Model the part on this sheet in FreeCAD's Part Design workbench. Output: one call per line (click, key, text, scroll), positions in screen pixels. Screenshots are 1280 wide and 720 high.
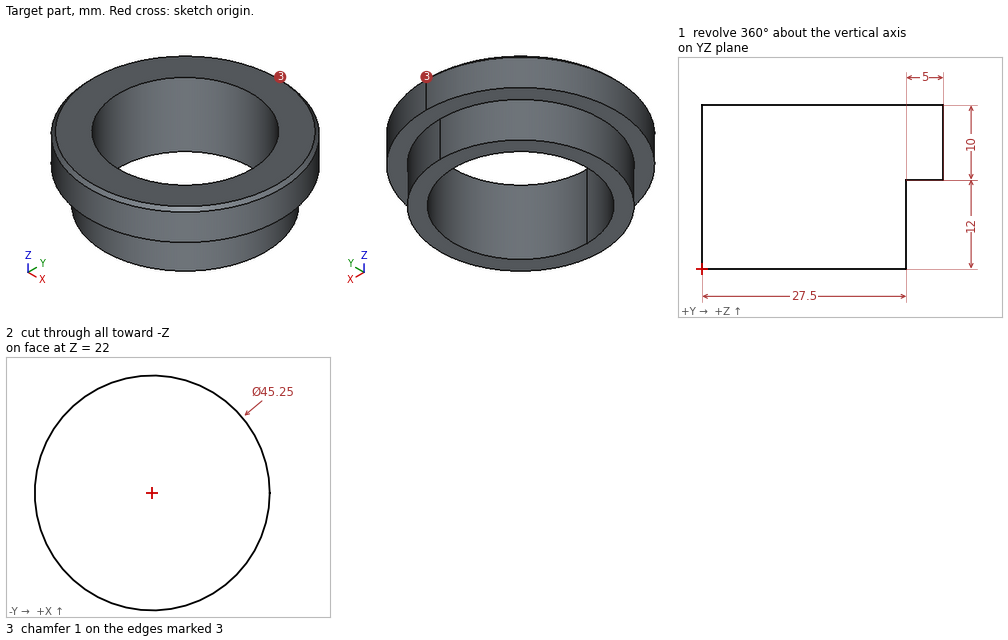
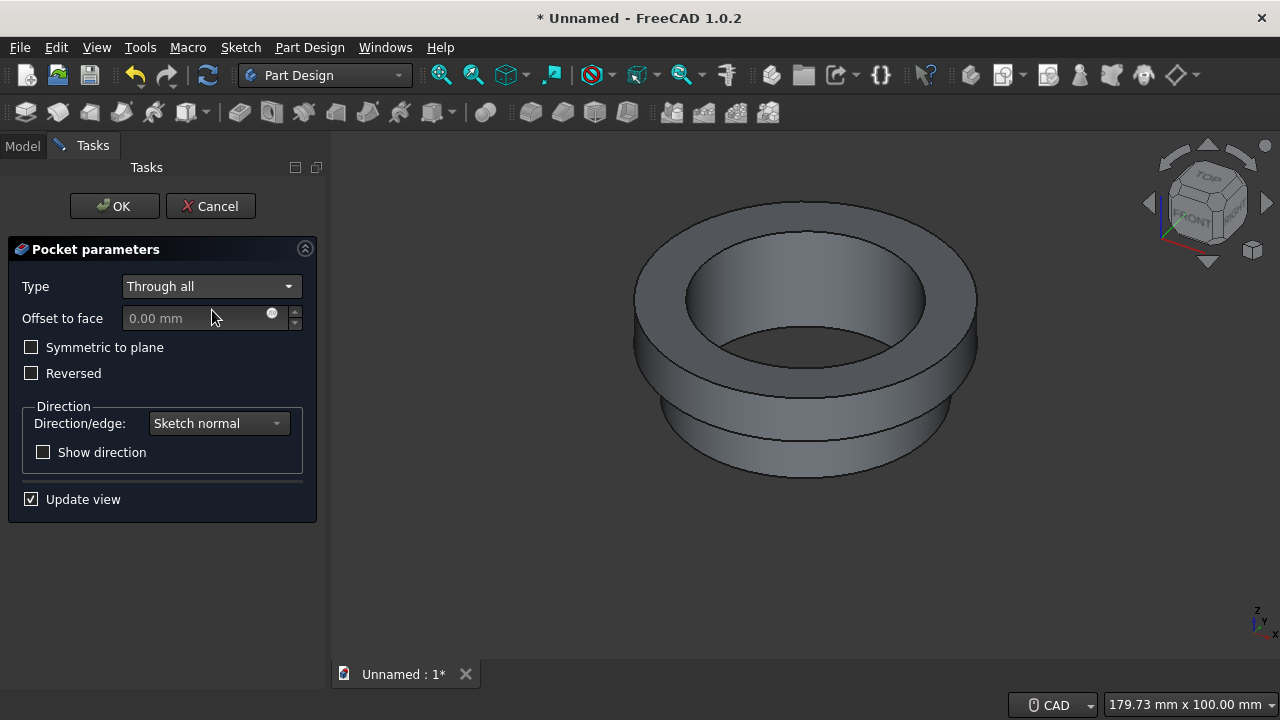
click(115, 206)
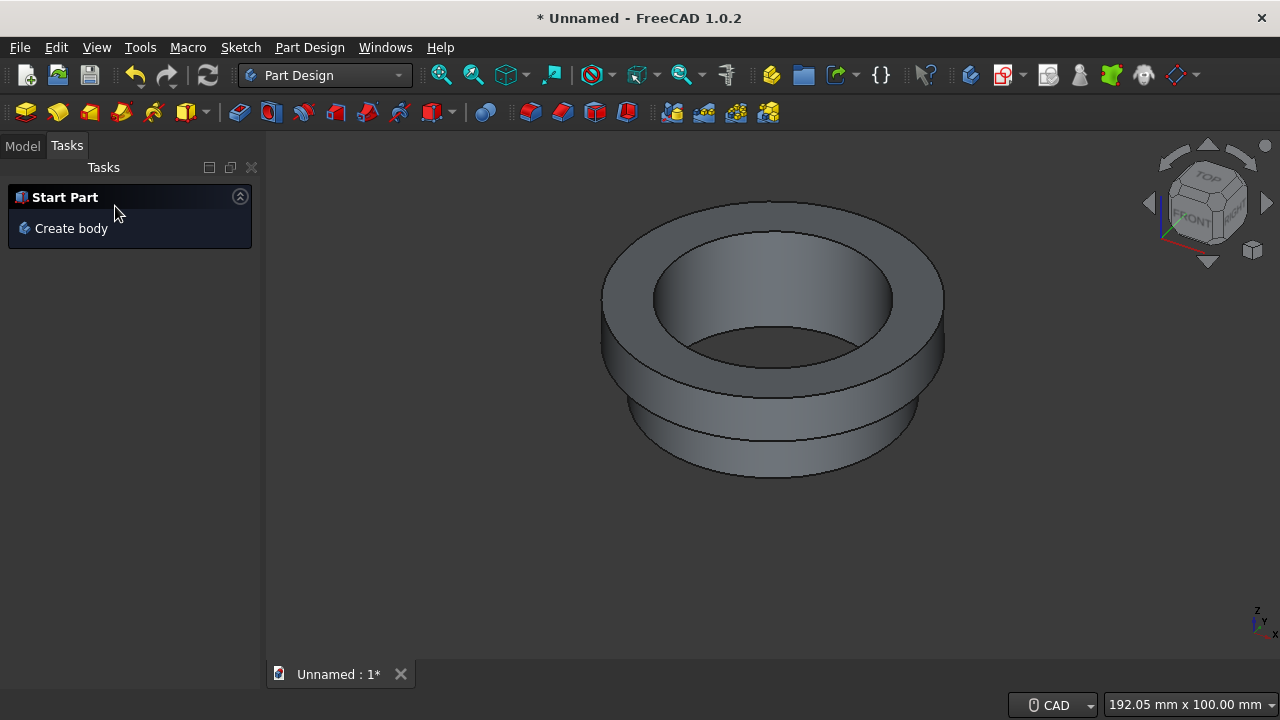
click(687, 384)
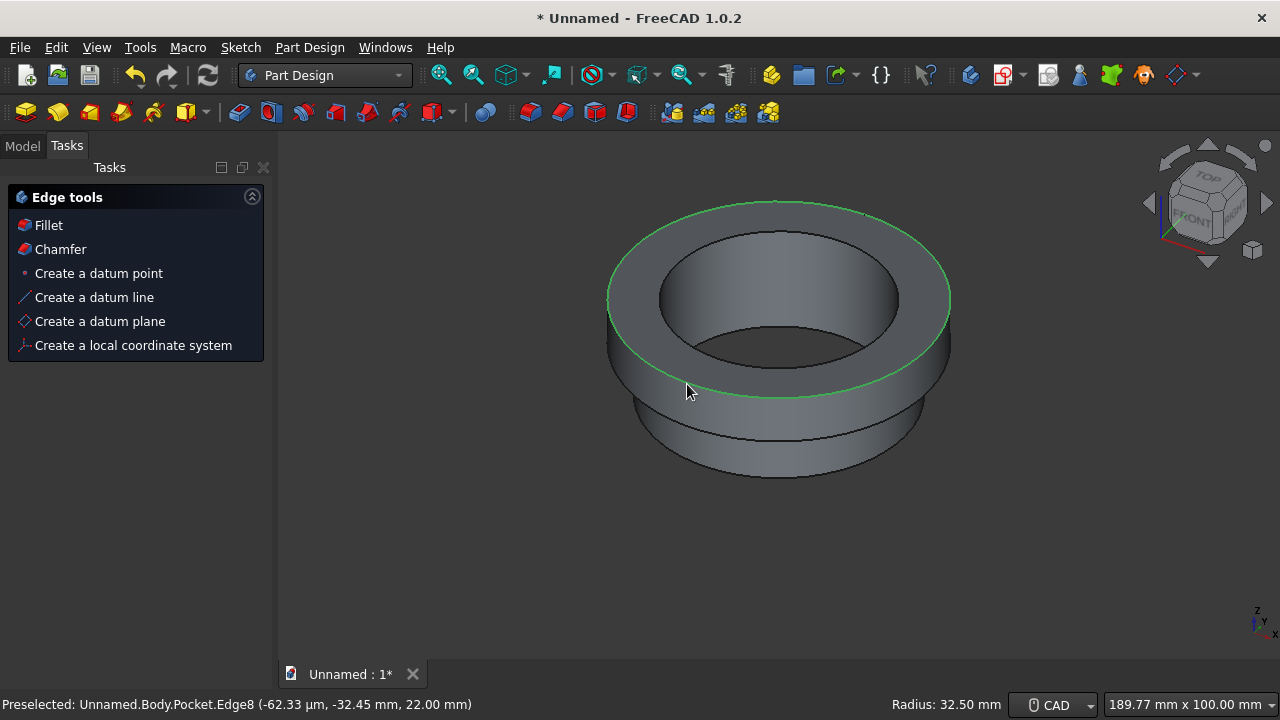
click(564, 112)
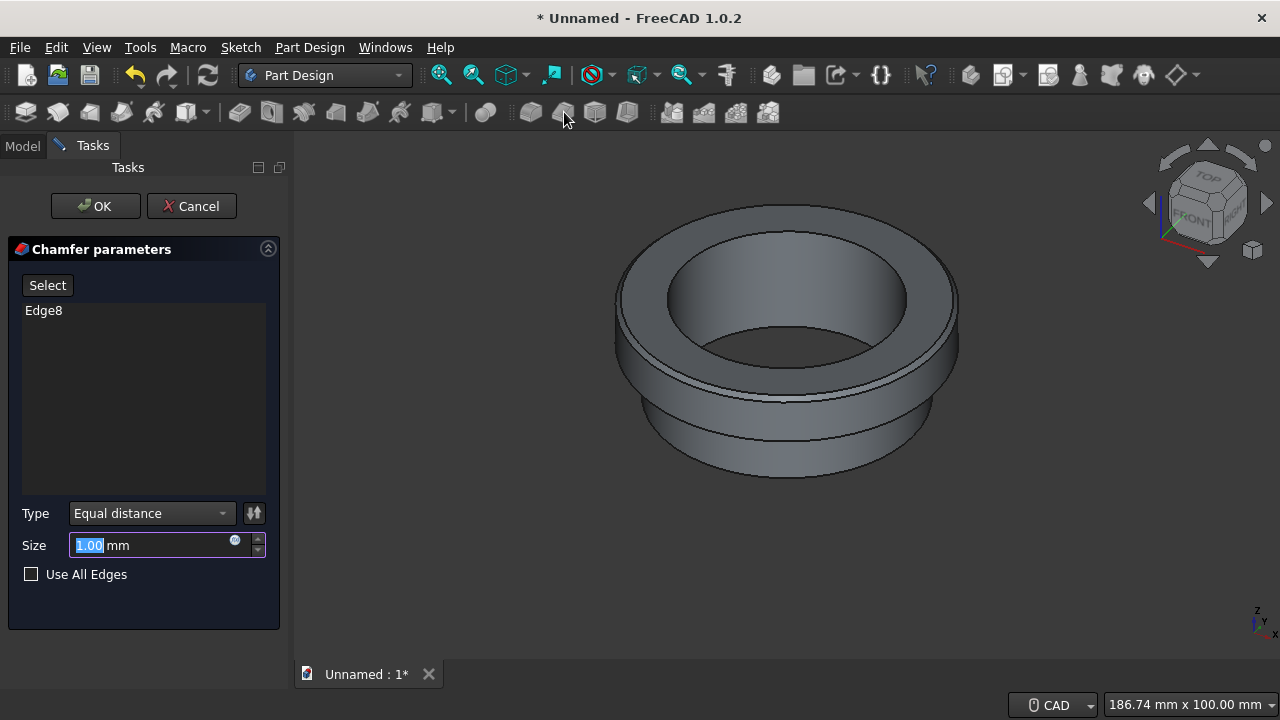
text(1)
key(Tab)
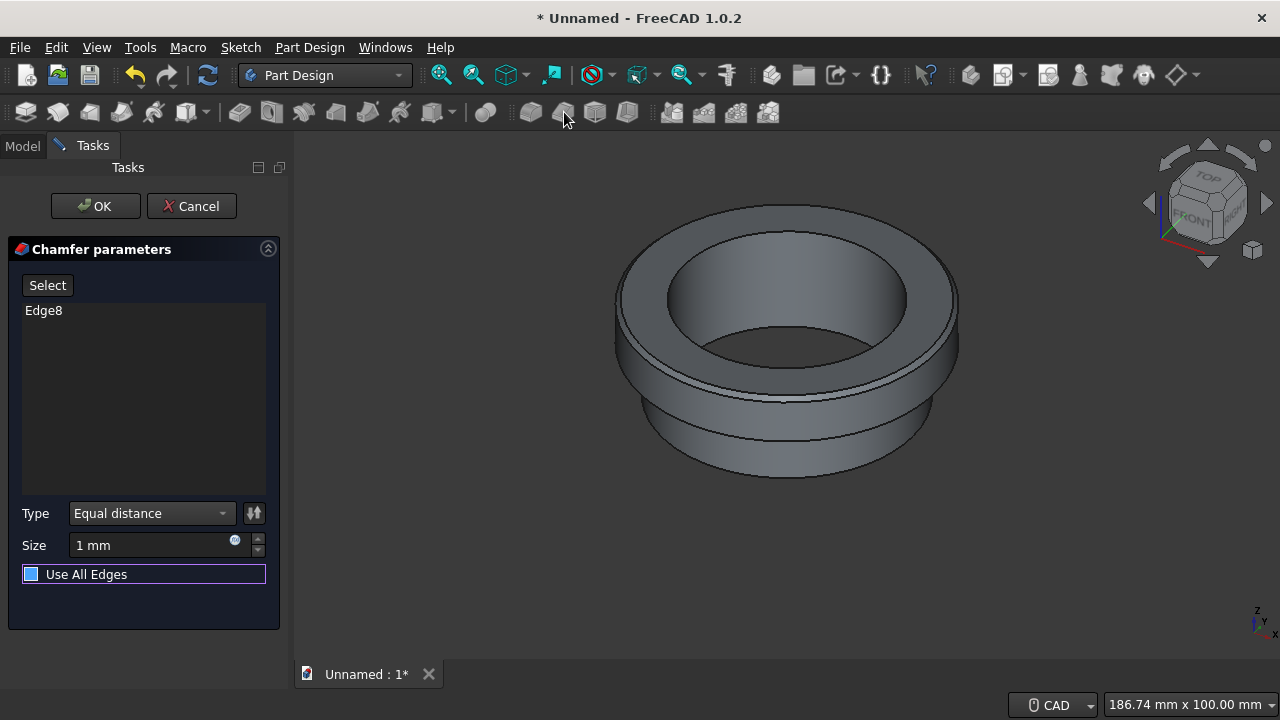
click(96, 206)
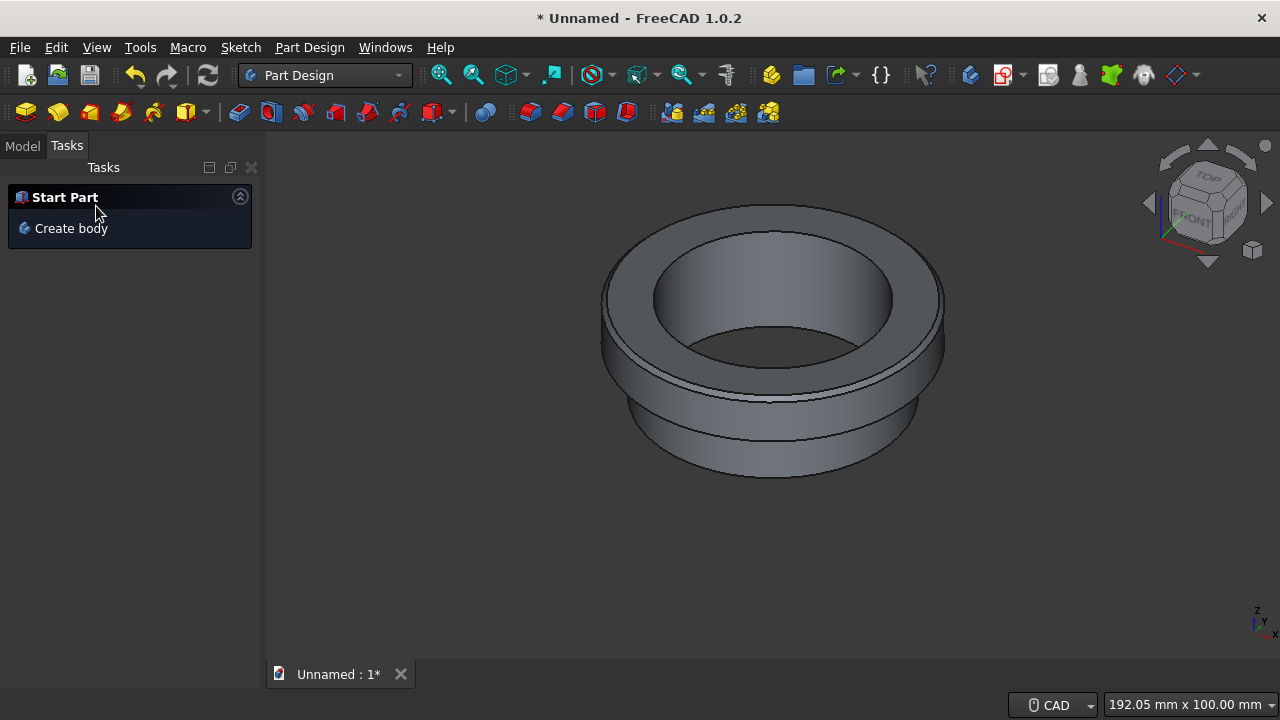
key(0)